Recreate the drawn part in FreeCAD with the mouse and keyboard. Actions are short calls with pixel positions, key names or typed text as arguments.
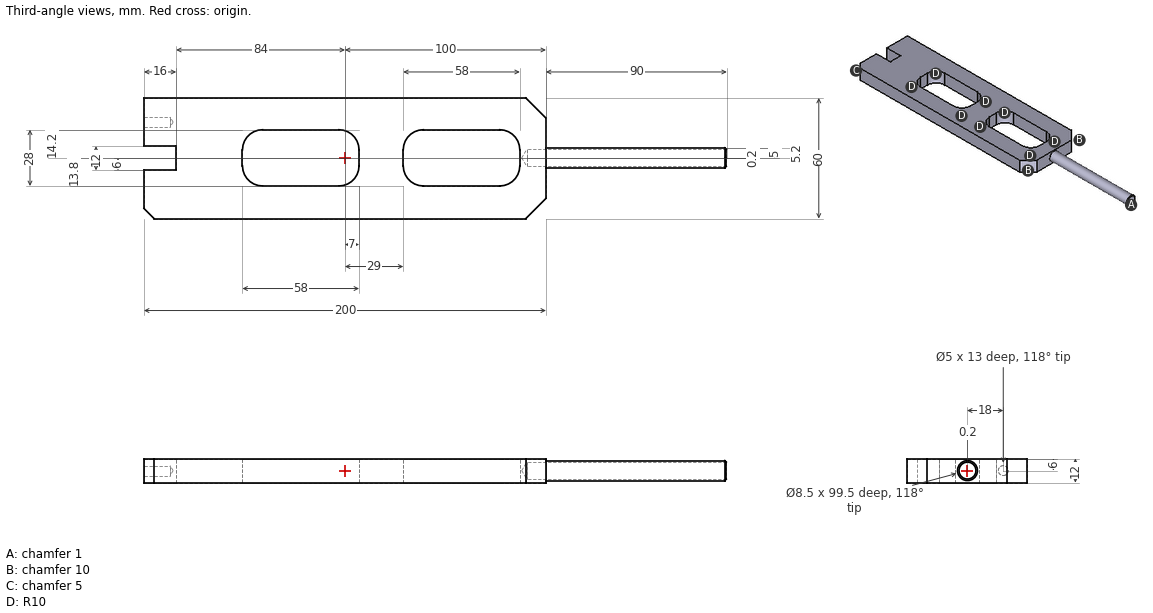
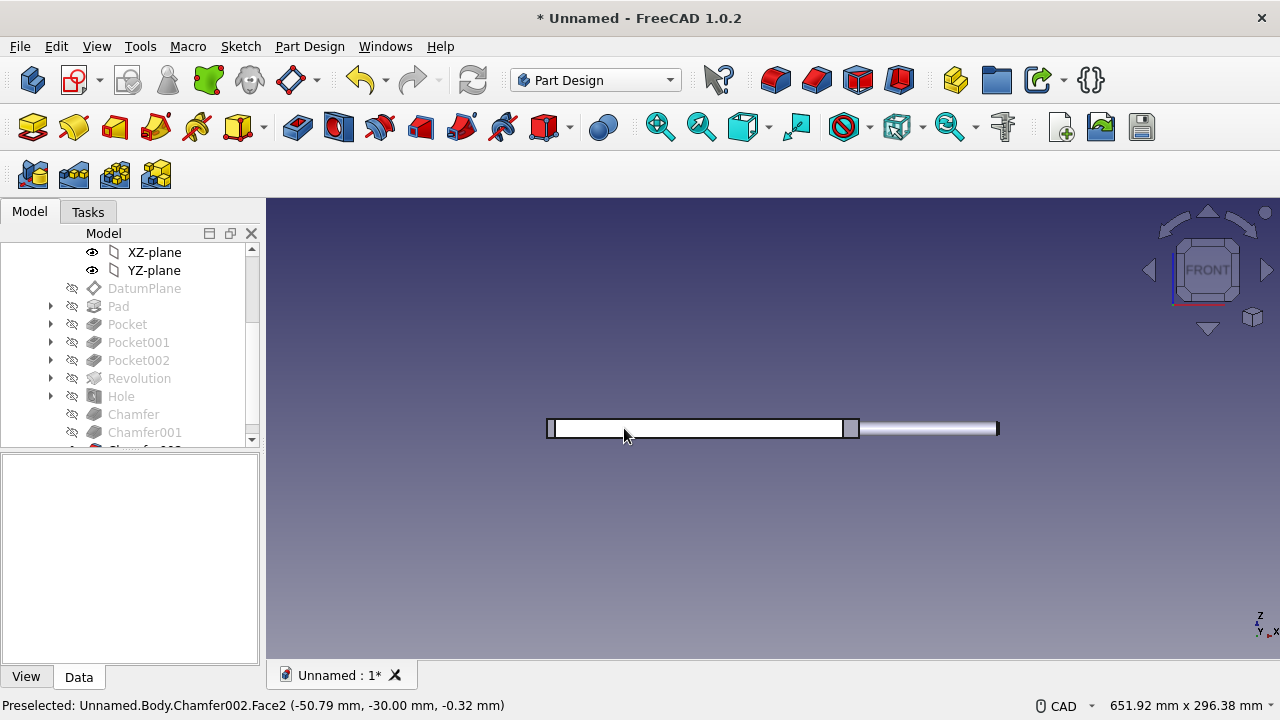
key(0)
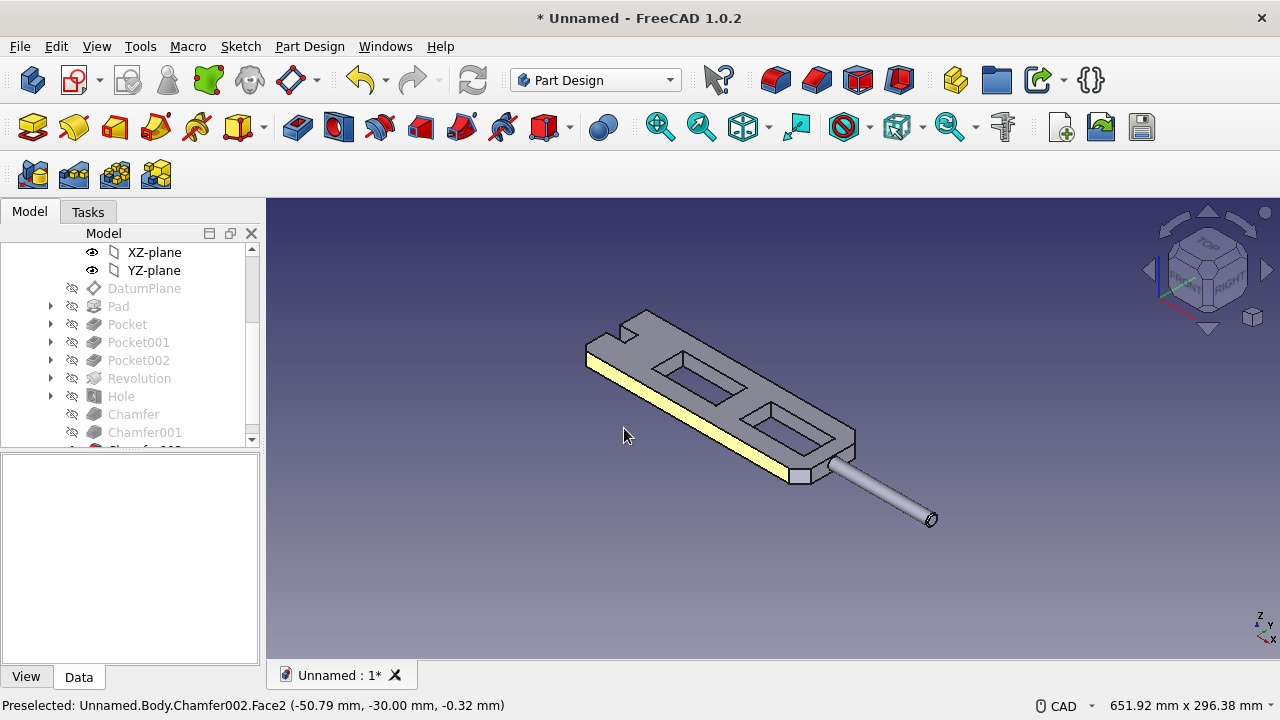
scroll(652, 375, up, 4)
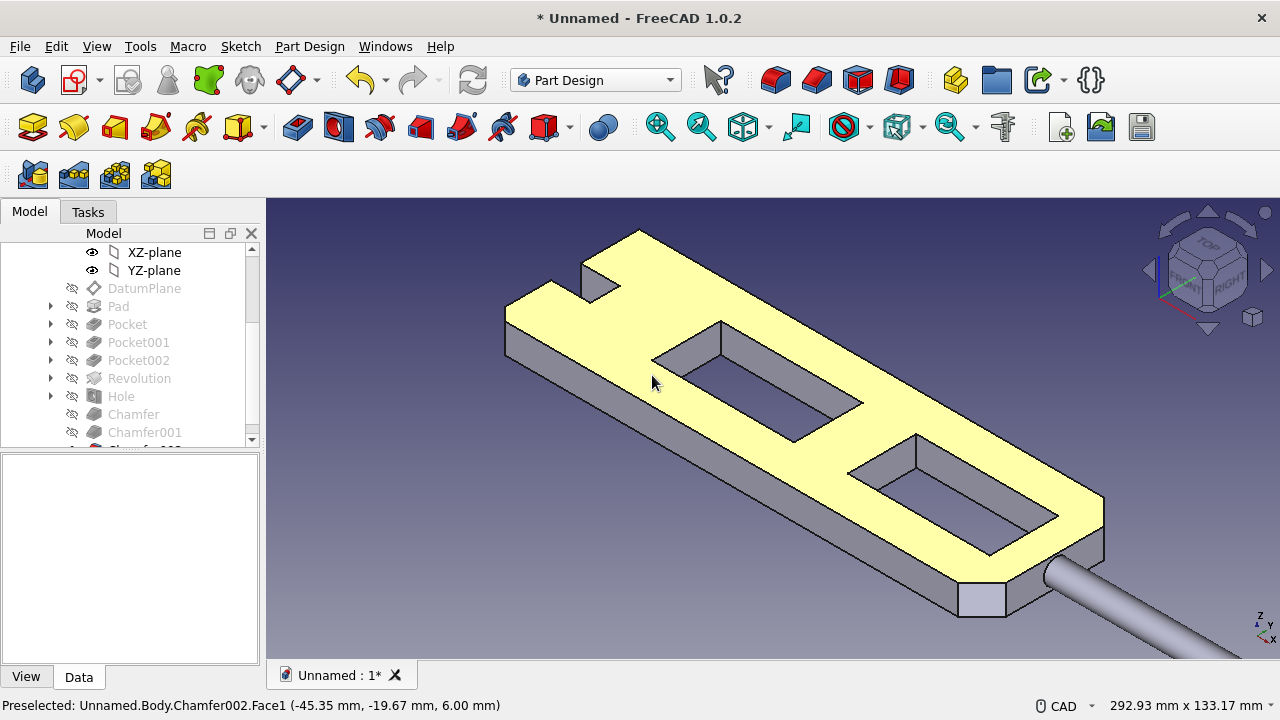
click(661, 128)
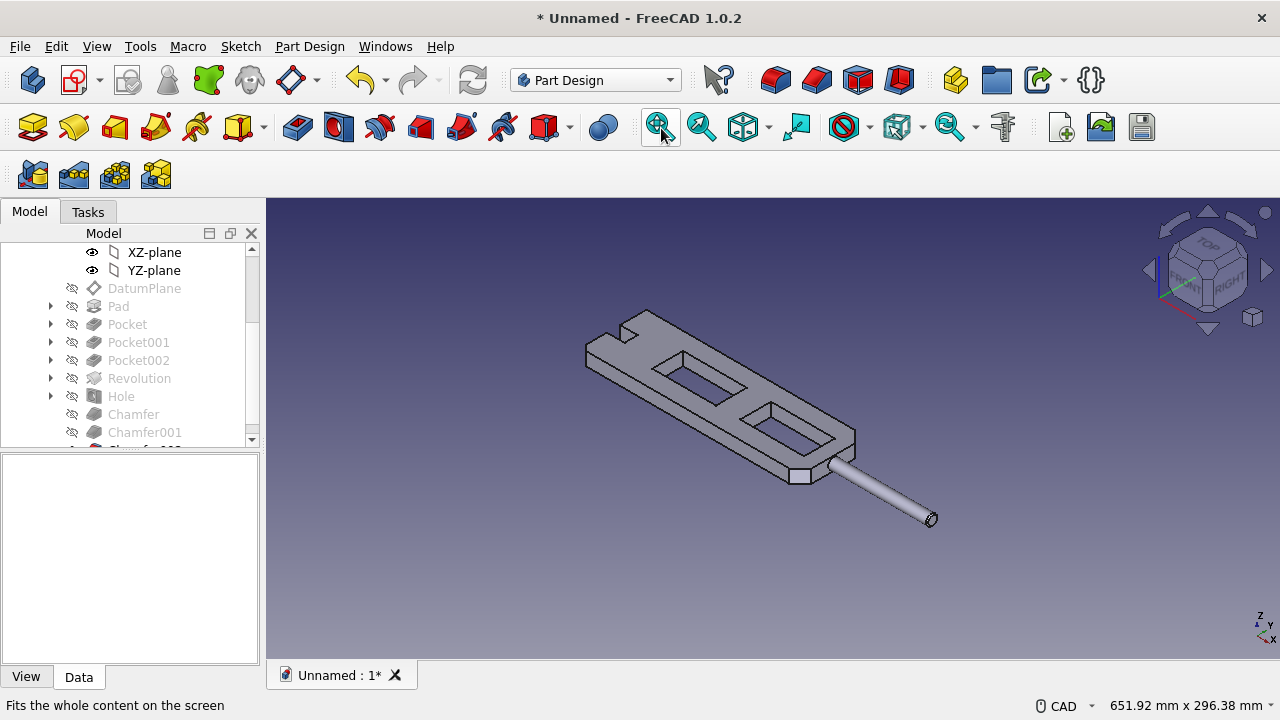
key(2)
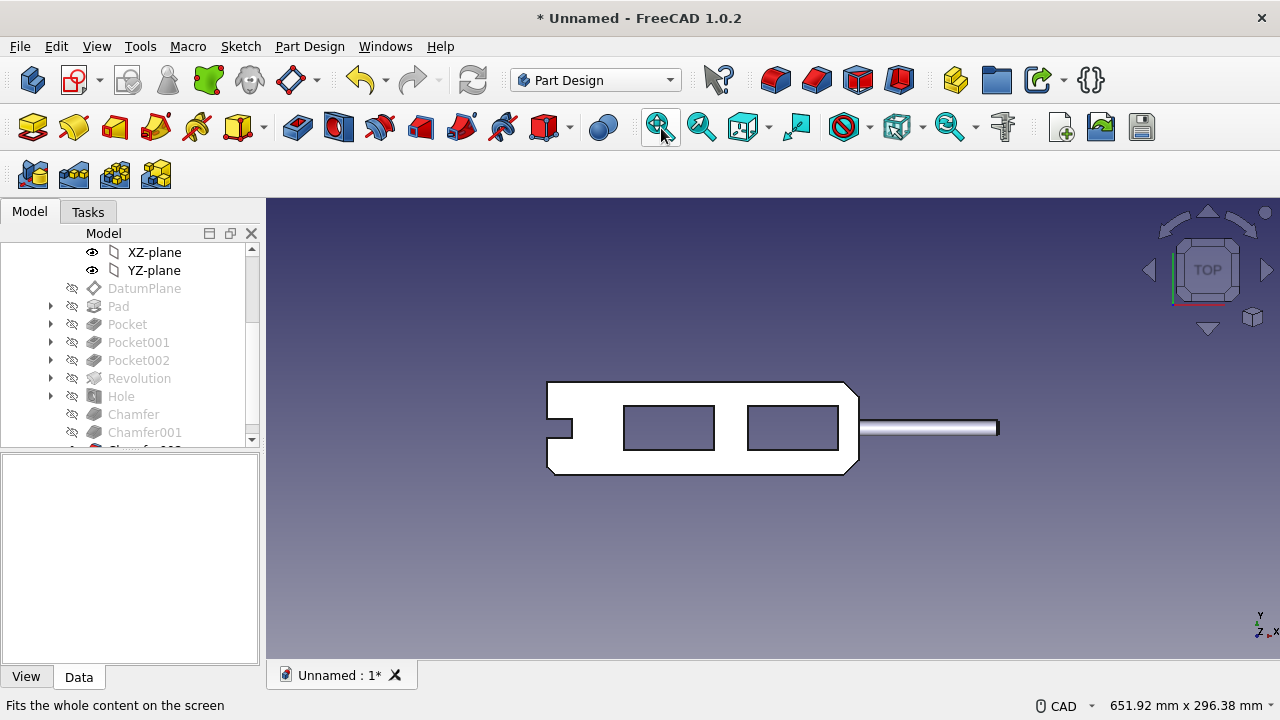
key(v)
key(f)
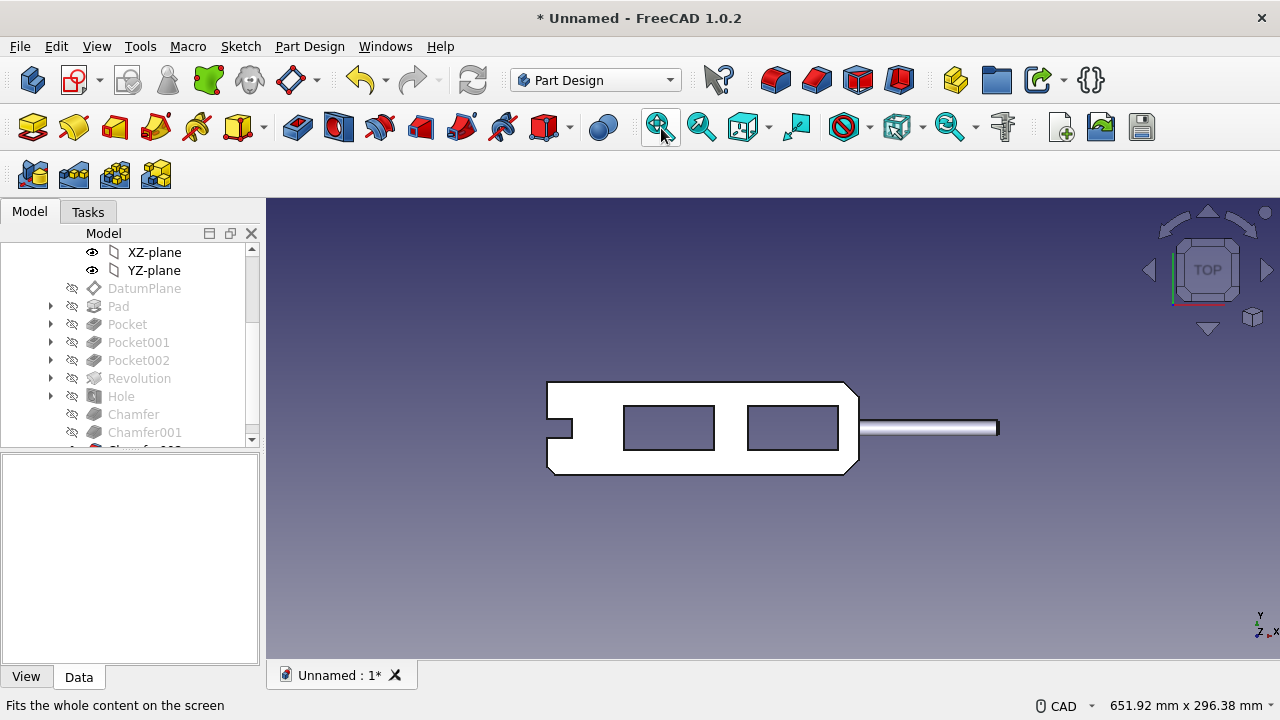
scroll(624, 449, up, 4)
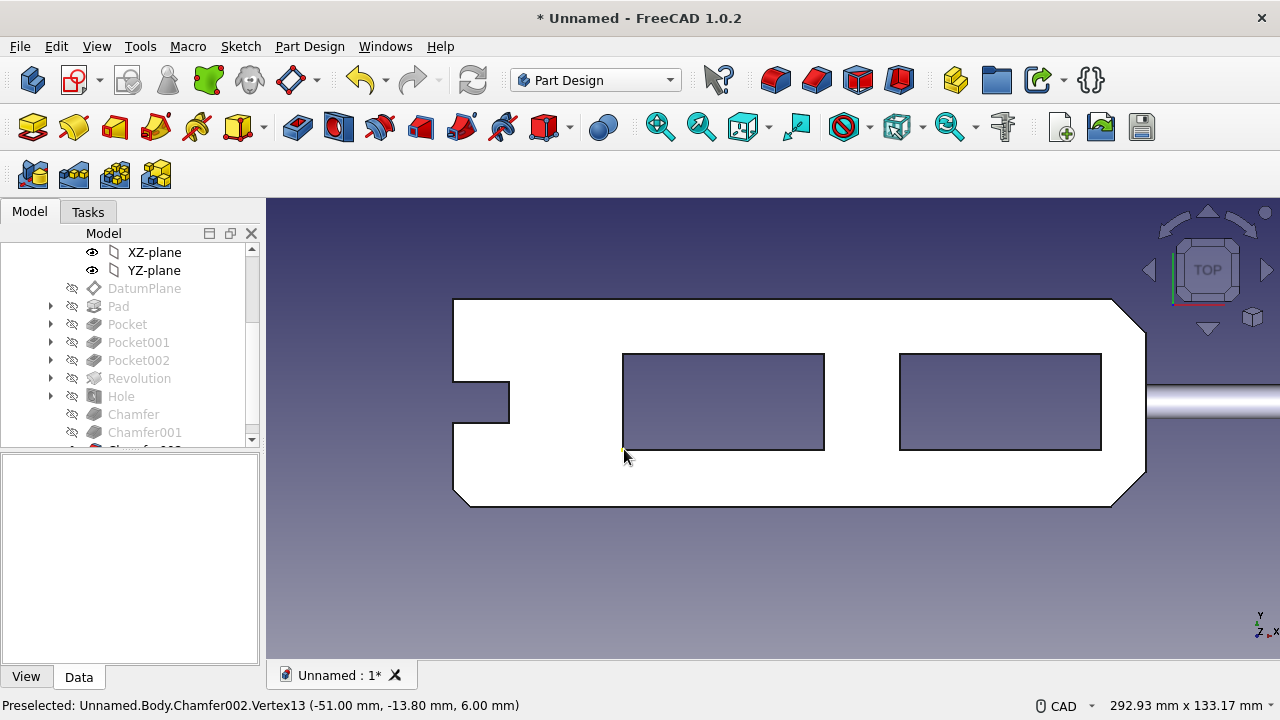
key(v)
key(f)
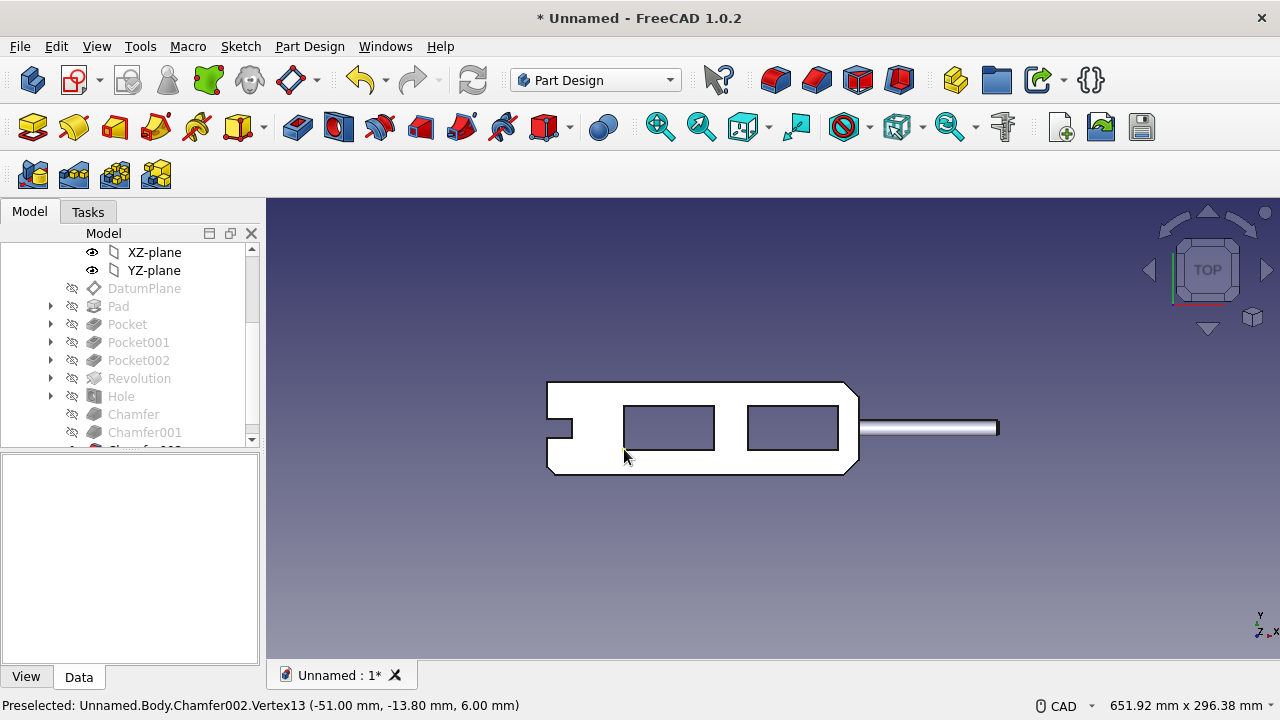
key(1)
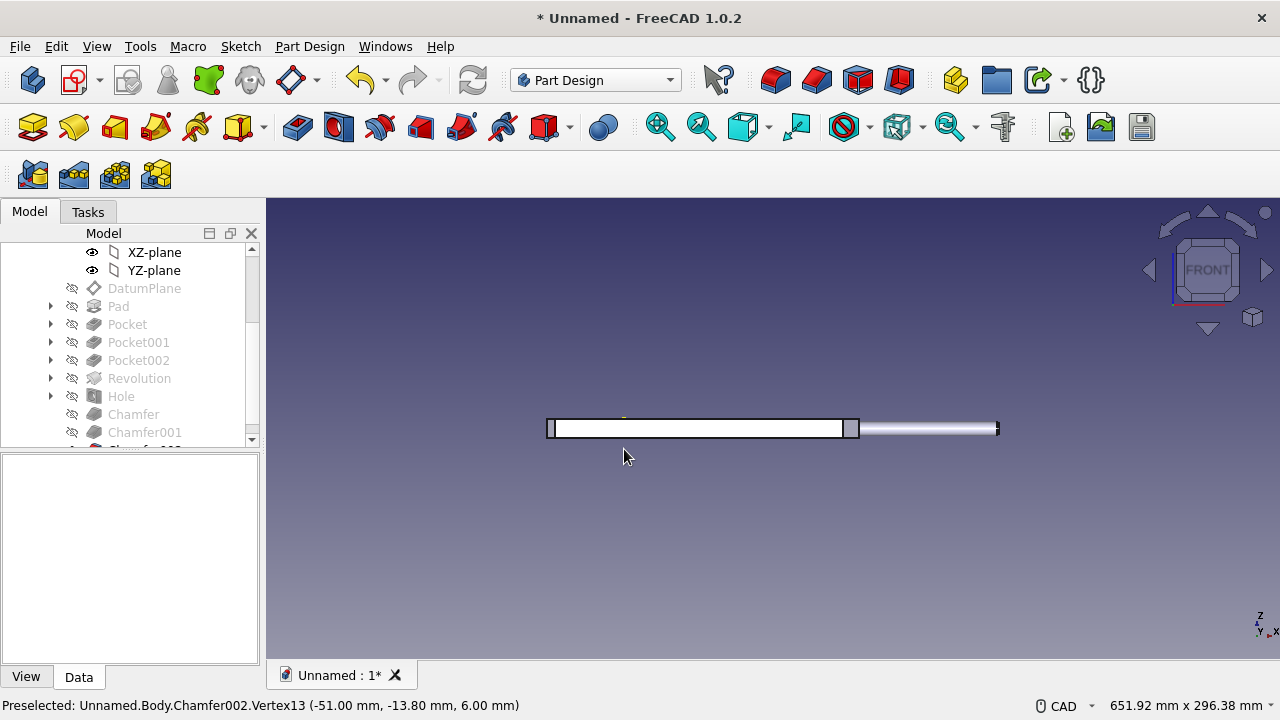
key(v)
key(f)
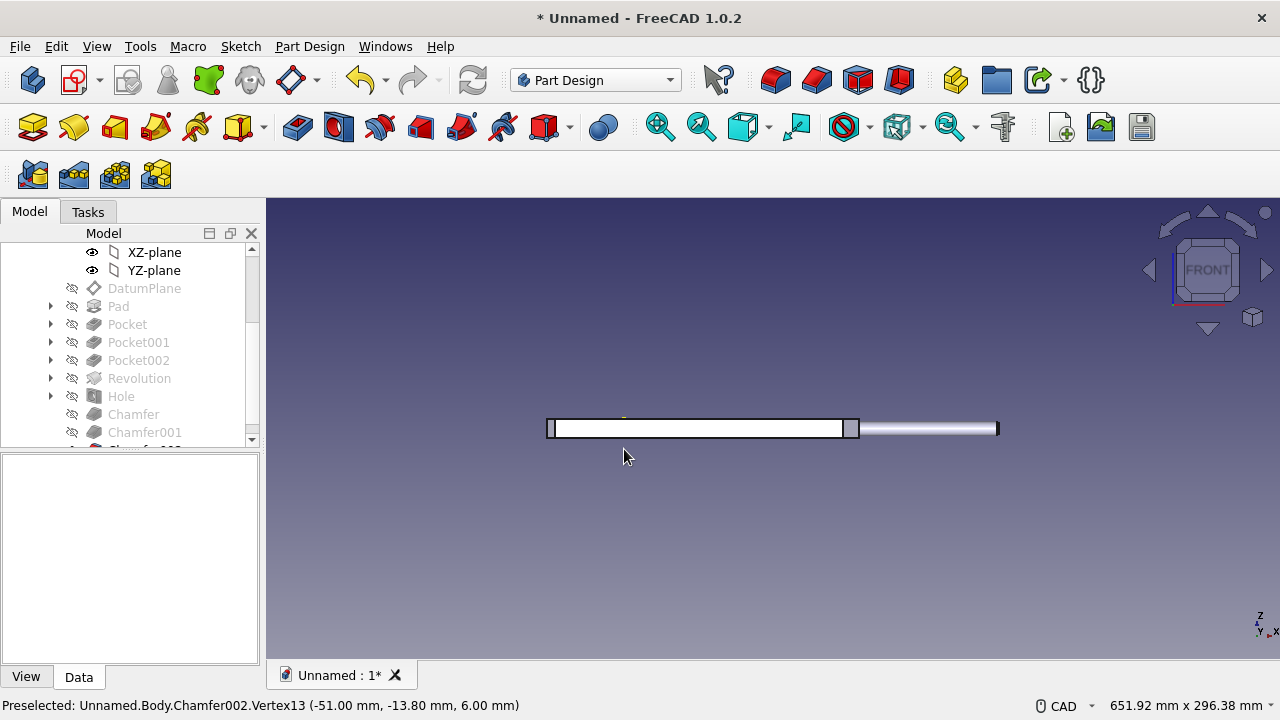
scroll(624, 428, up, 4)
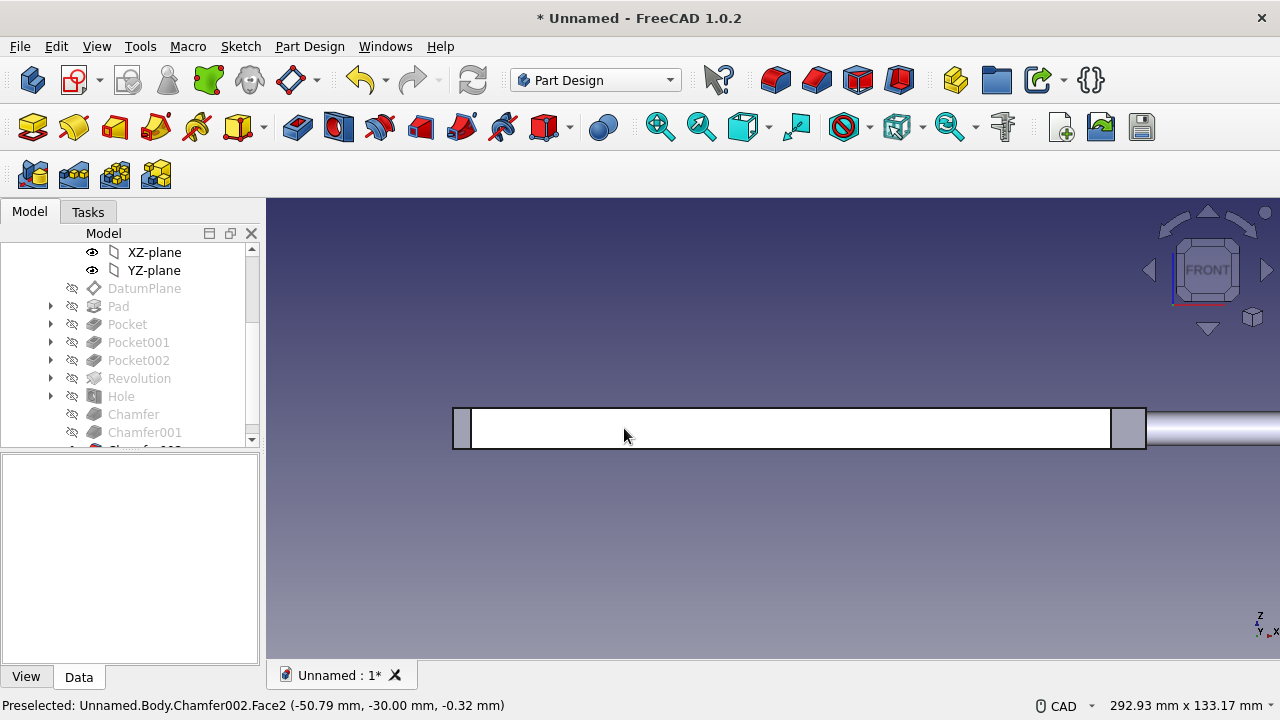
key(v)
key(f)